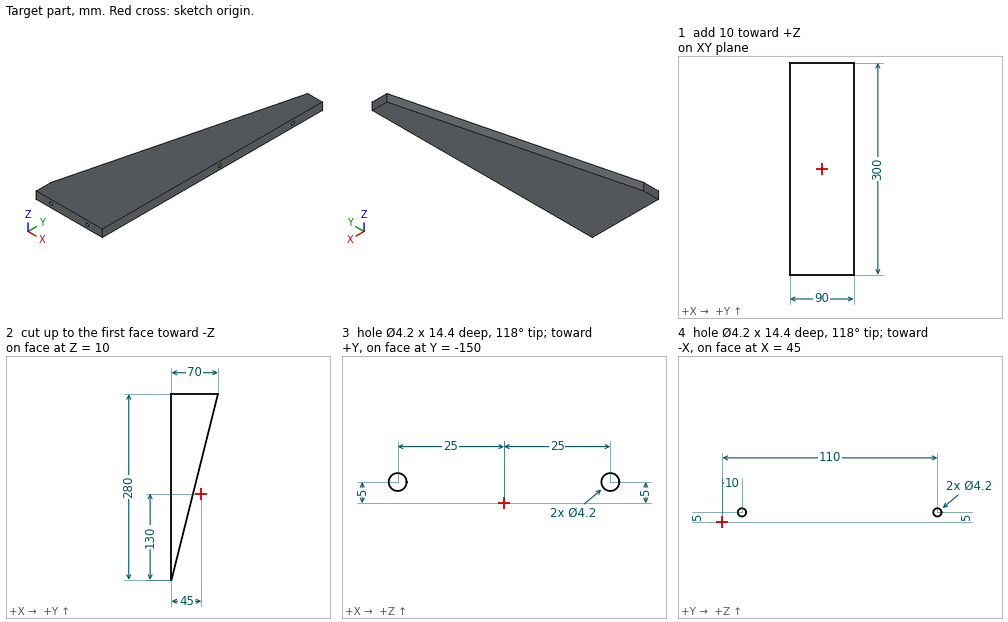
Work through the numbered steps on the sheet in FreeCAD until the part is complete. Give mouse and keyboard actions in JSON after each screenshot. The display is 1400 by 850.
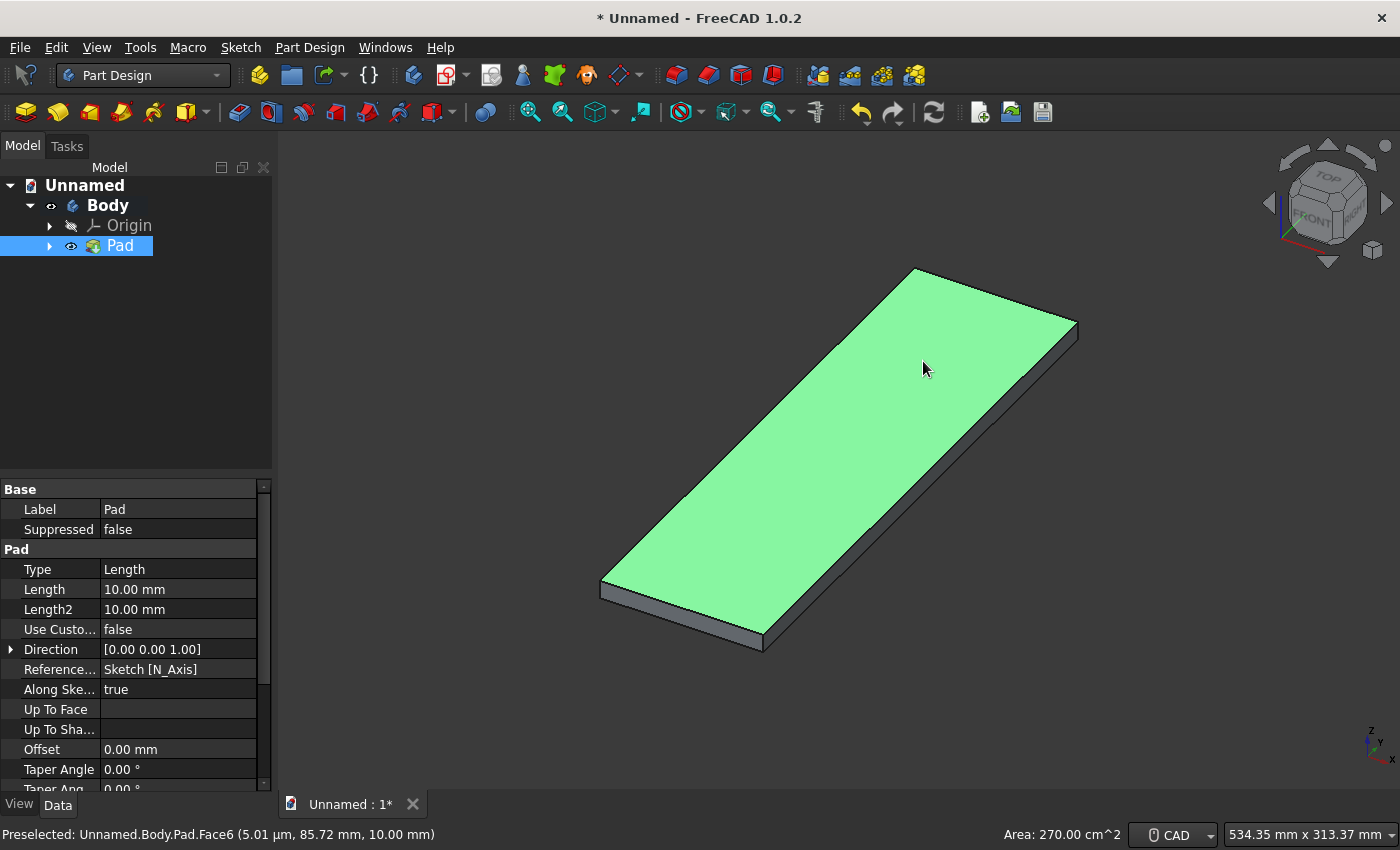
{"action": "left_click", "coordinate": [446, 76]}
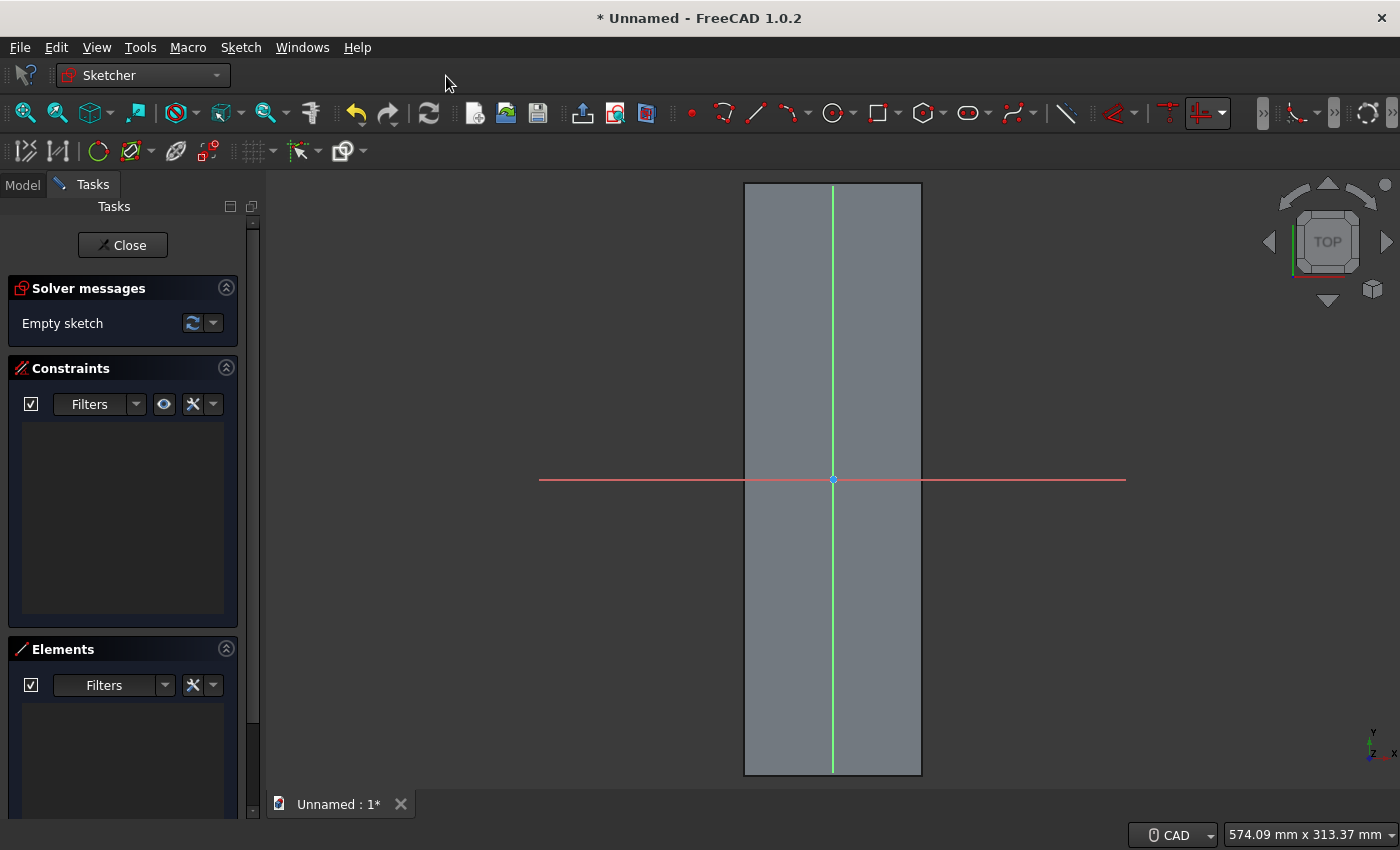
{"action": "scroll", "coordinate": [665, 520], "scroll_direction": "down", "scroll_amount": 2}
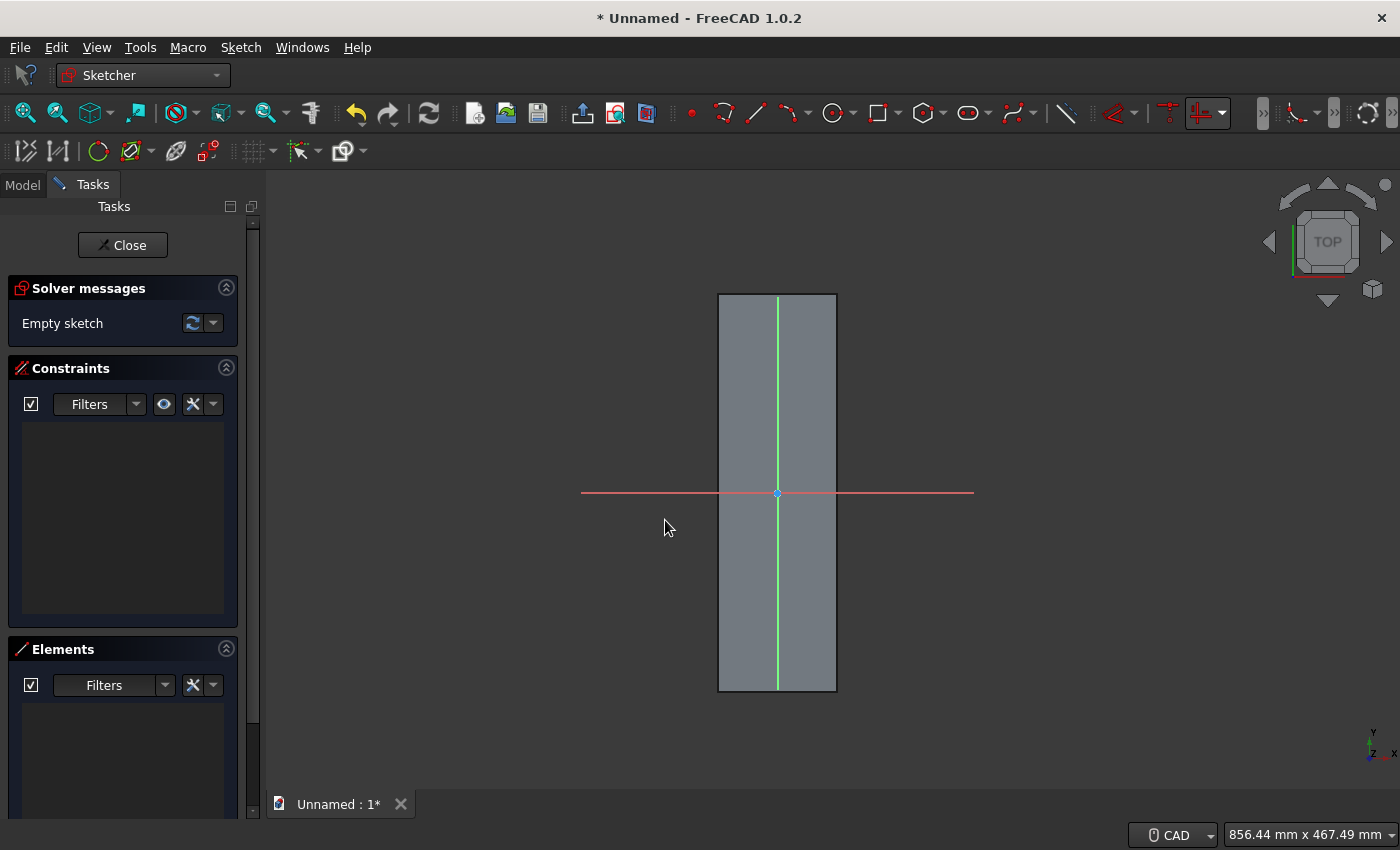
{"action": "key", "text": "g m"}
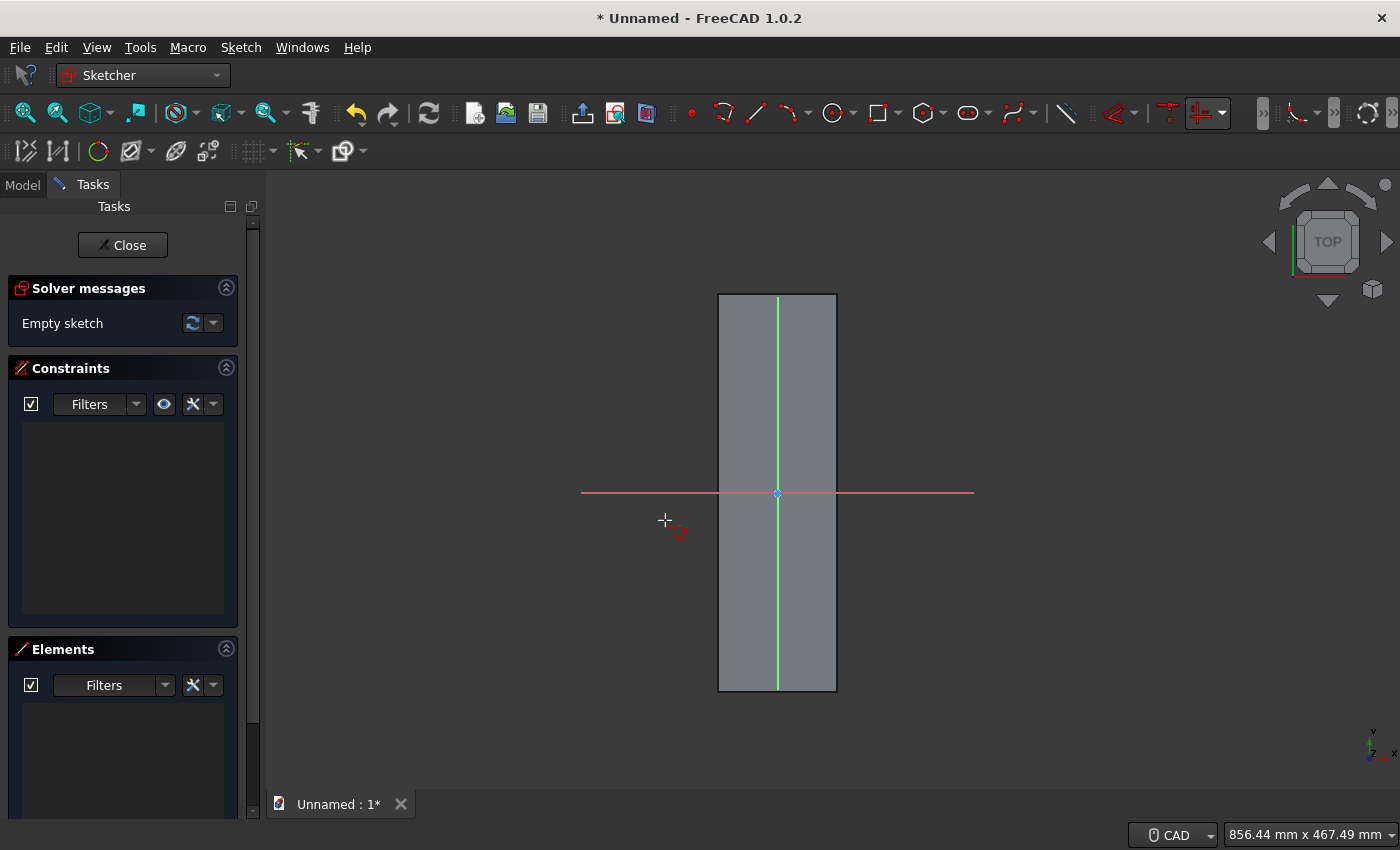
{"action": "left_click", "coordinate": [718, 665]}
{"action": "left_click", "coordinate": [811, 294]}
{"action": "left_click", "coordinate": [718, 294]}
{"action": "left_click", "coordinate": [718, 666]}
{"action": "key", "text": "Escape"}
{"action": "key", "text": "Escape"}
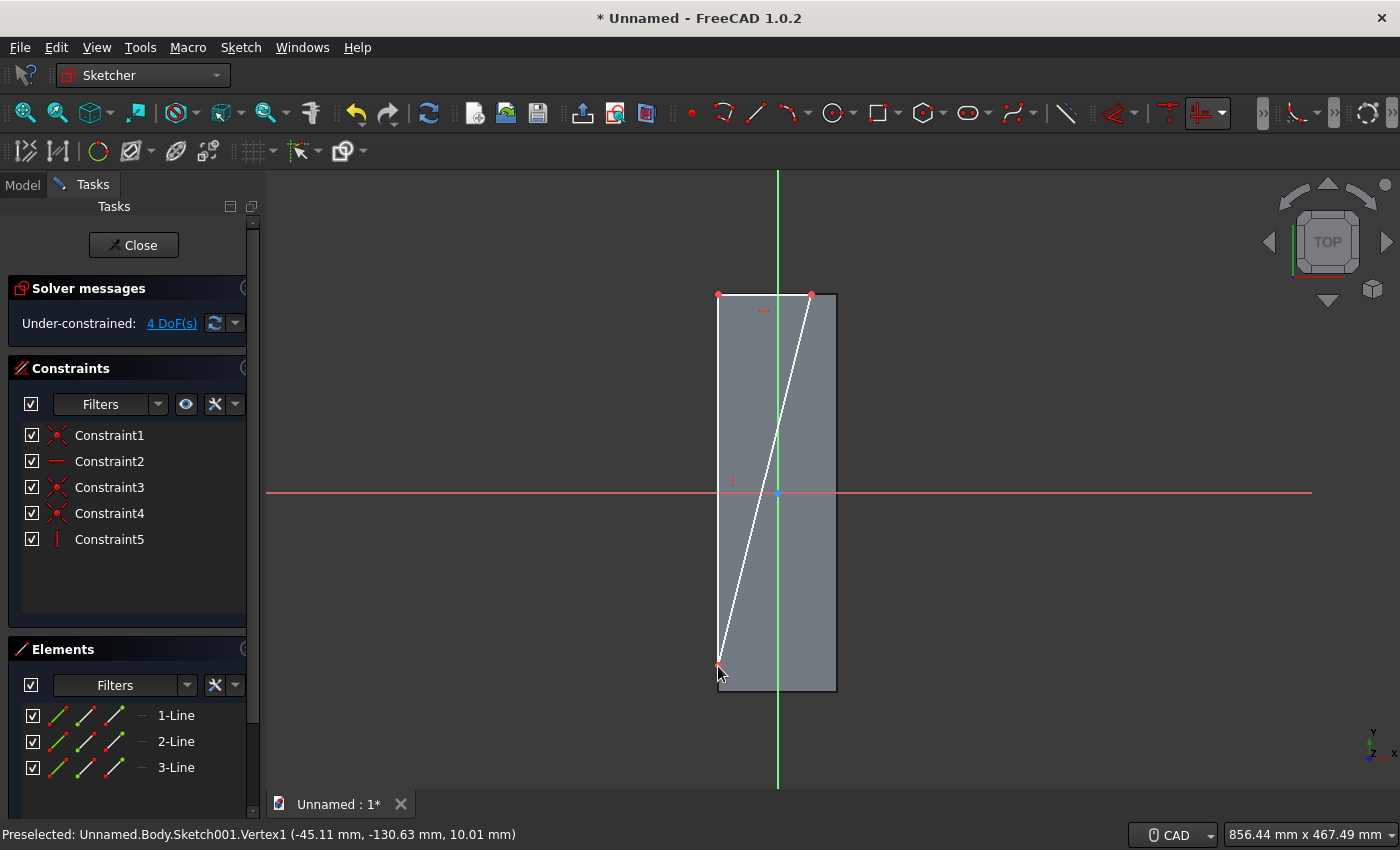
{"action": "left_click", "coordinate": [1114, 114]}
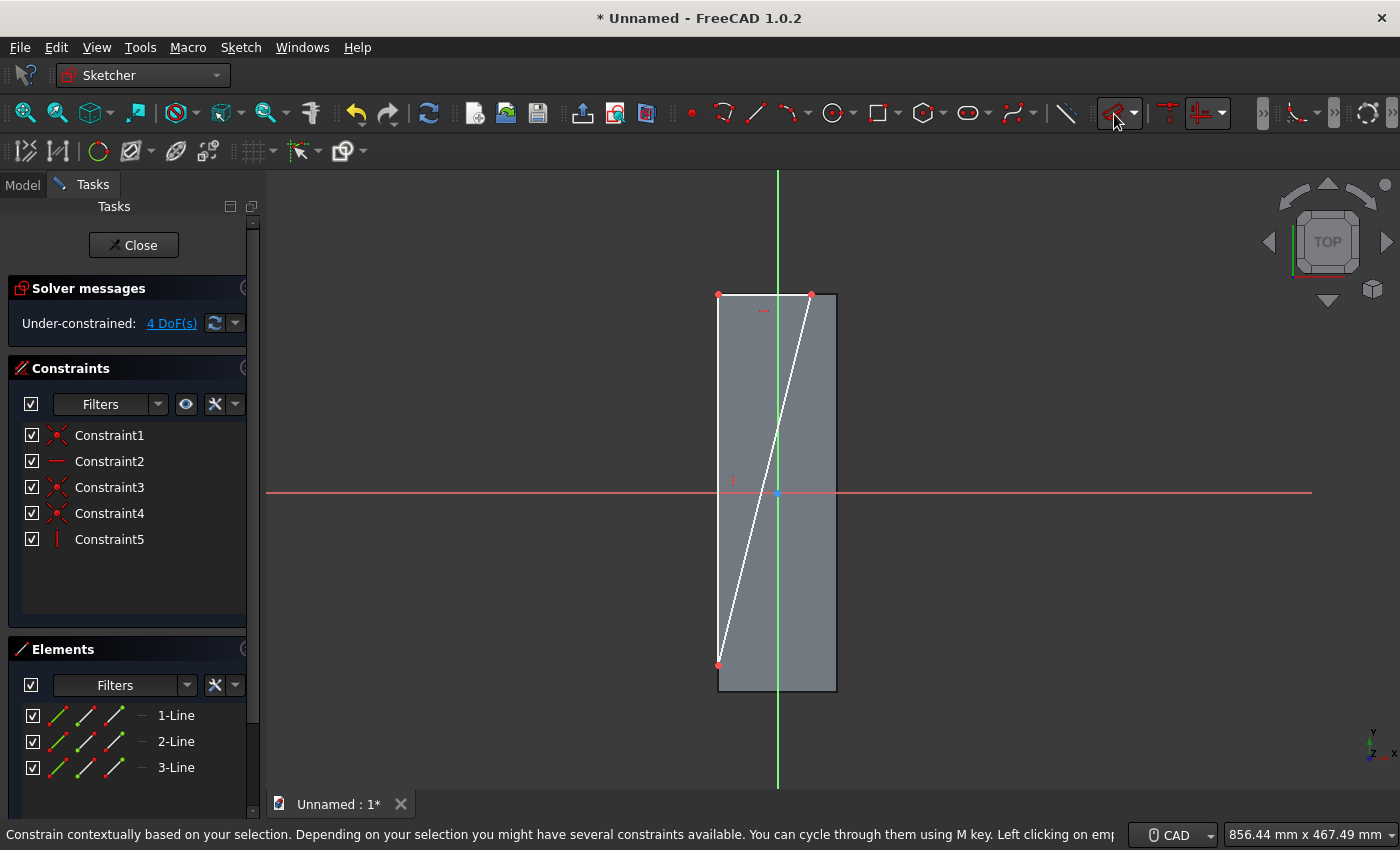
{"action": "left_click", "coordinate": [746, 295]}
{"action": "left_click", "coordinate": [765, 261]}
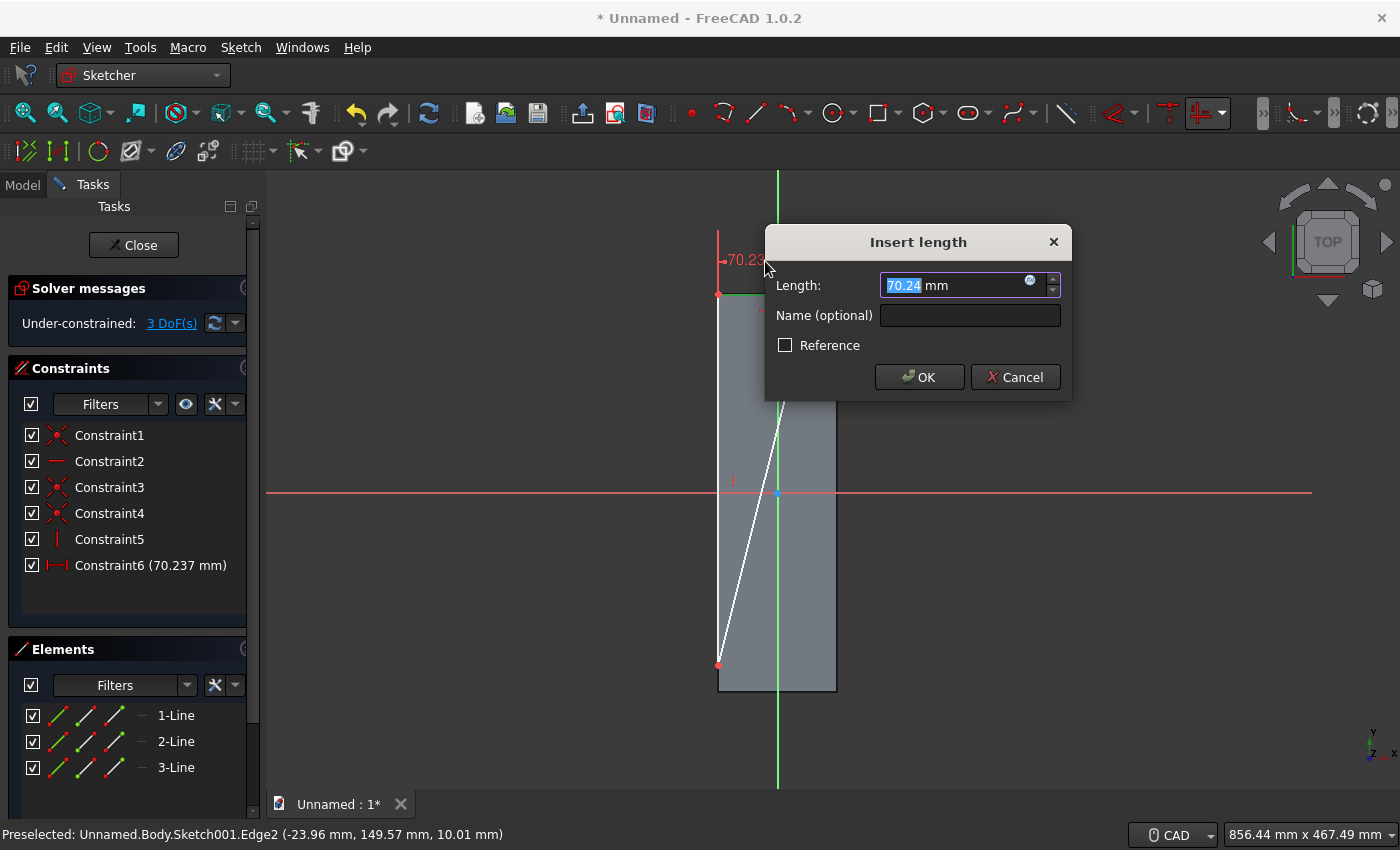
{"action": "type", "text": "70"}
{"action": "key", "text": "Return"}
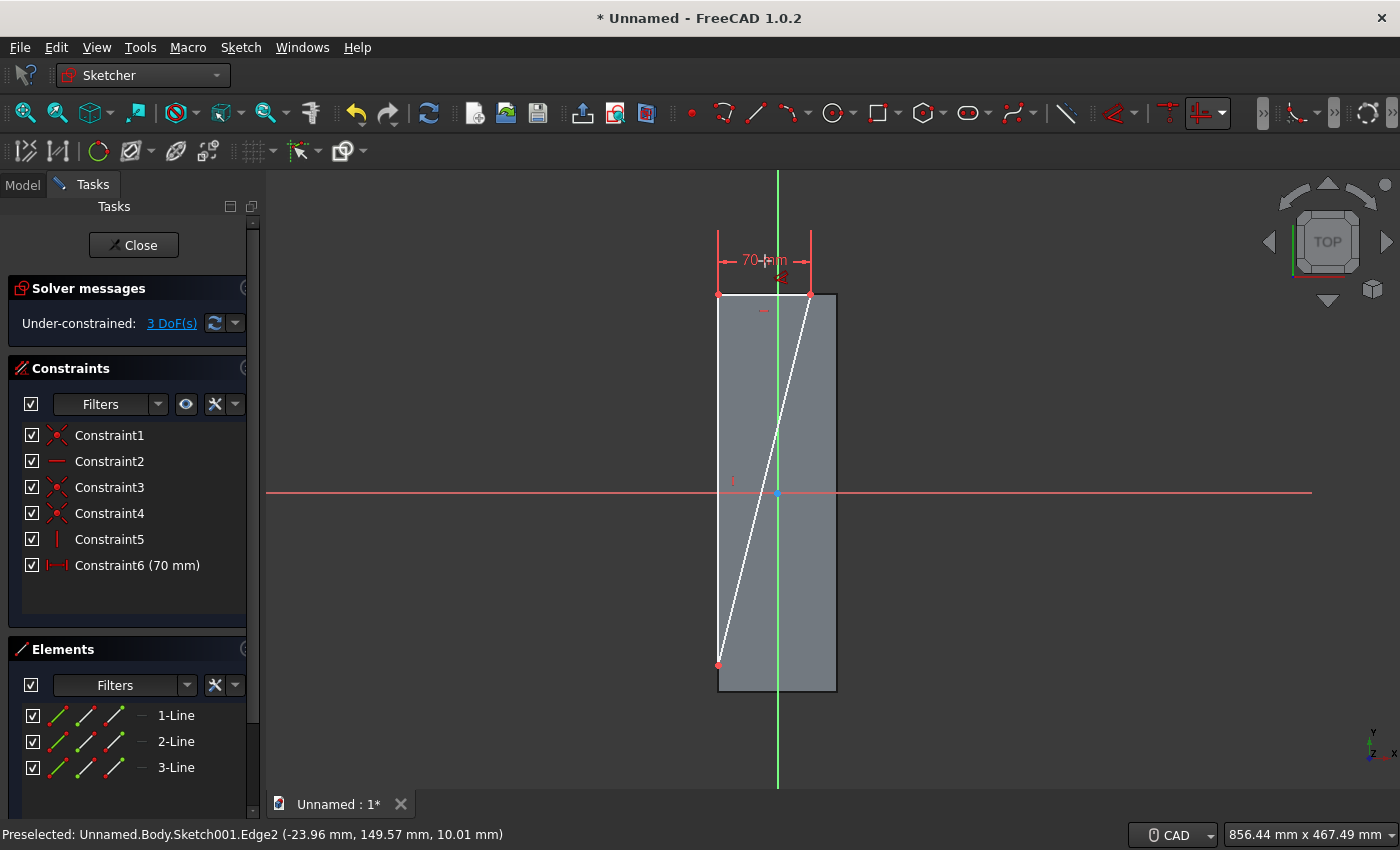
{"action": "left_click", "coordinate": [718, 406]}
{"action": "left_click", "coordinate": [684, 395]}